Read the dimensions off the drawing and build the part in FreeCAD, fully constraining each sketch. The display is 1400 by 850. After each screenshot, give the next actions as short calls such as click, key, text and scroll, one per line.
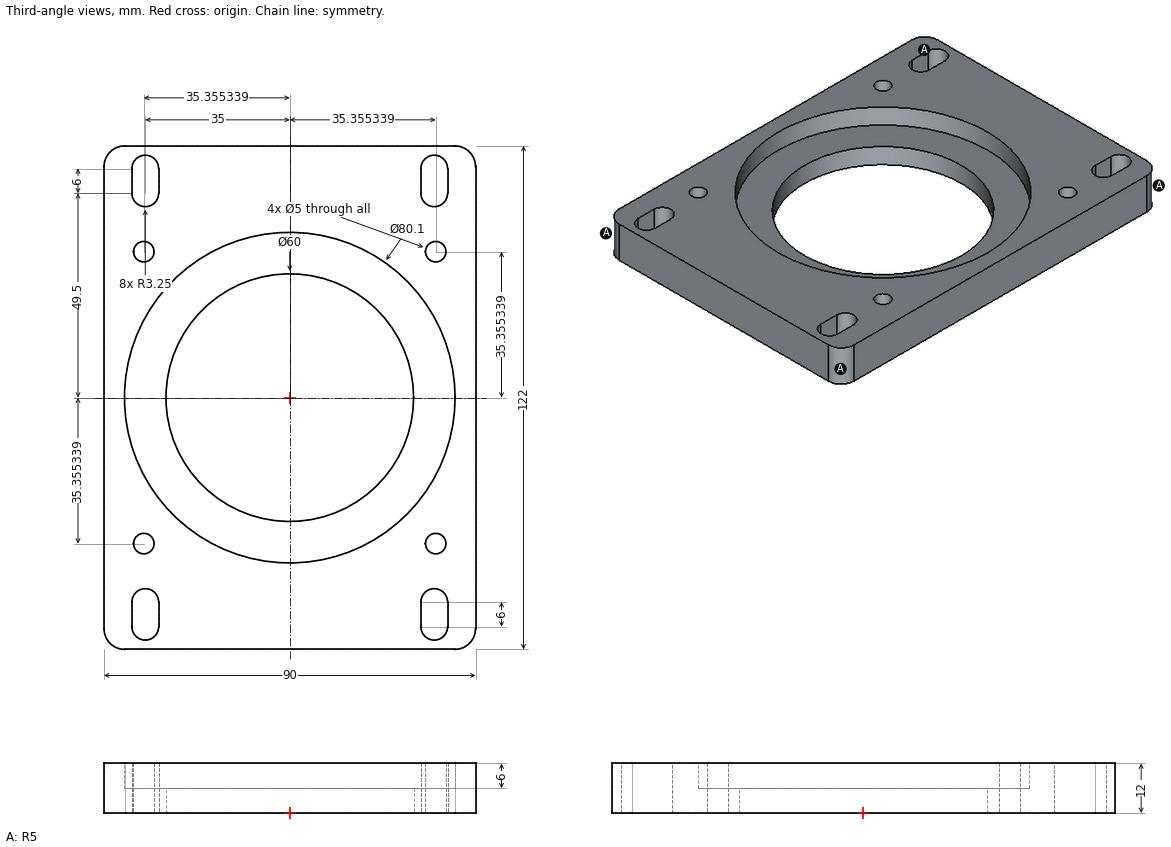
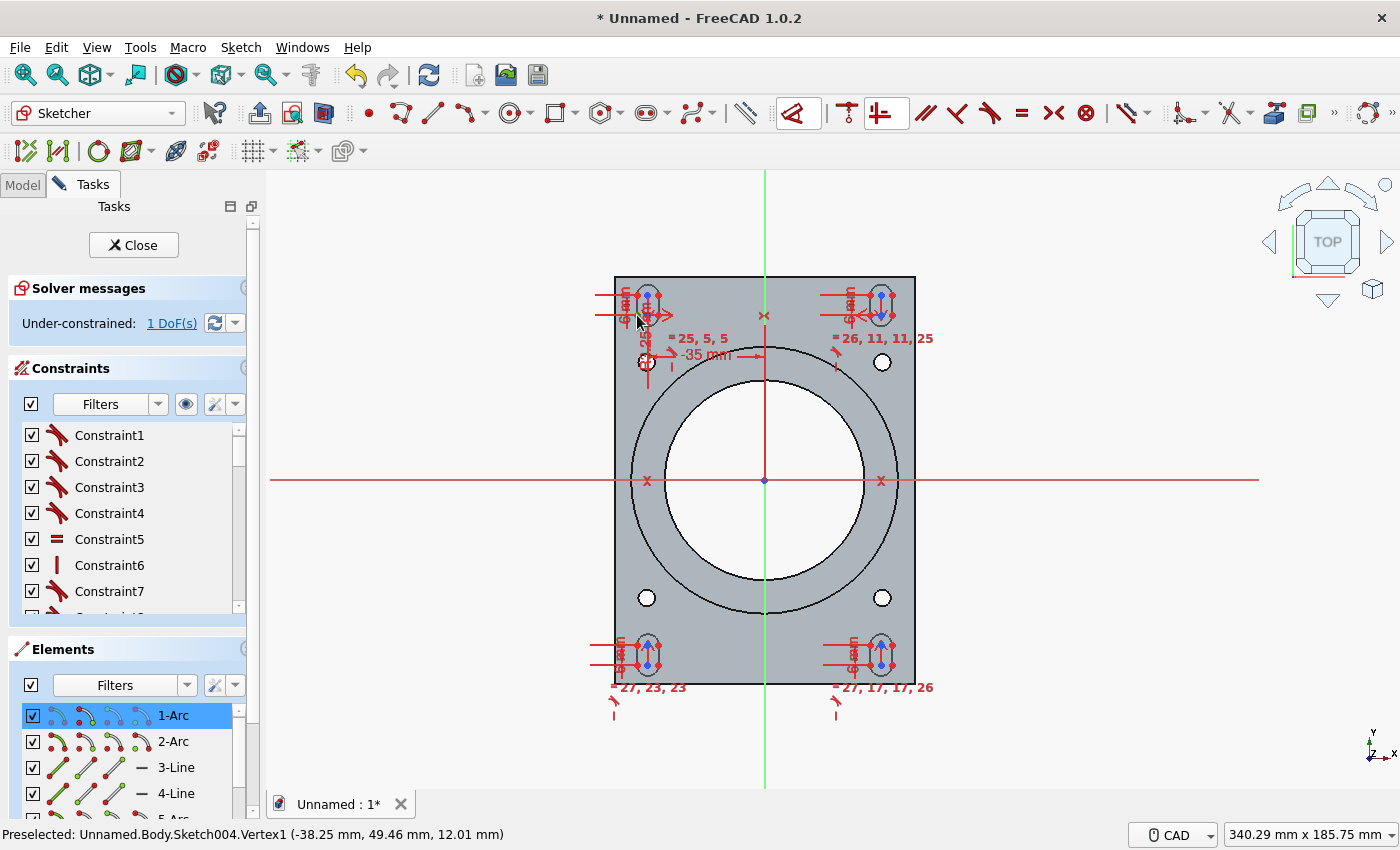
click(816, 114)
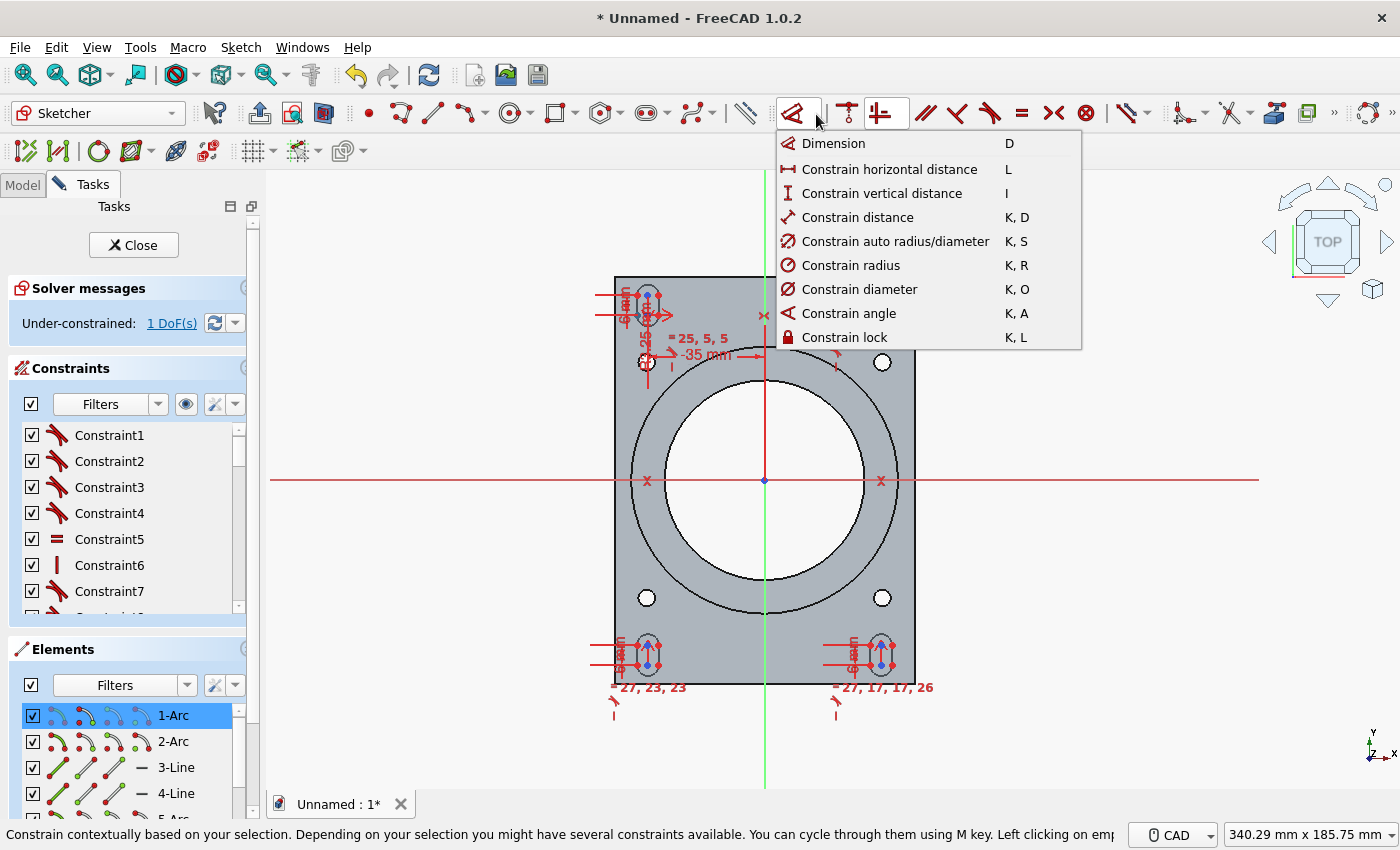
click(929, 193)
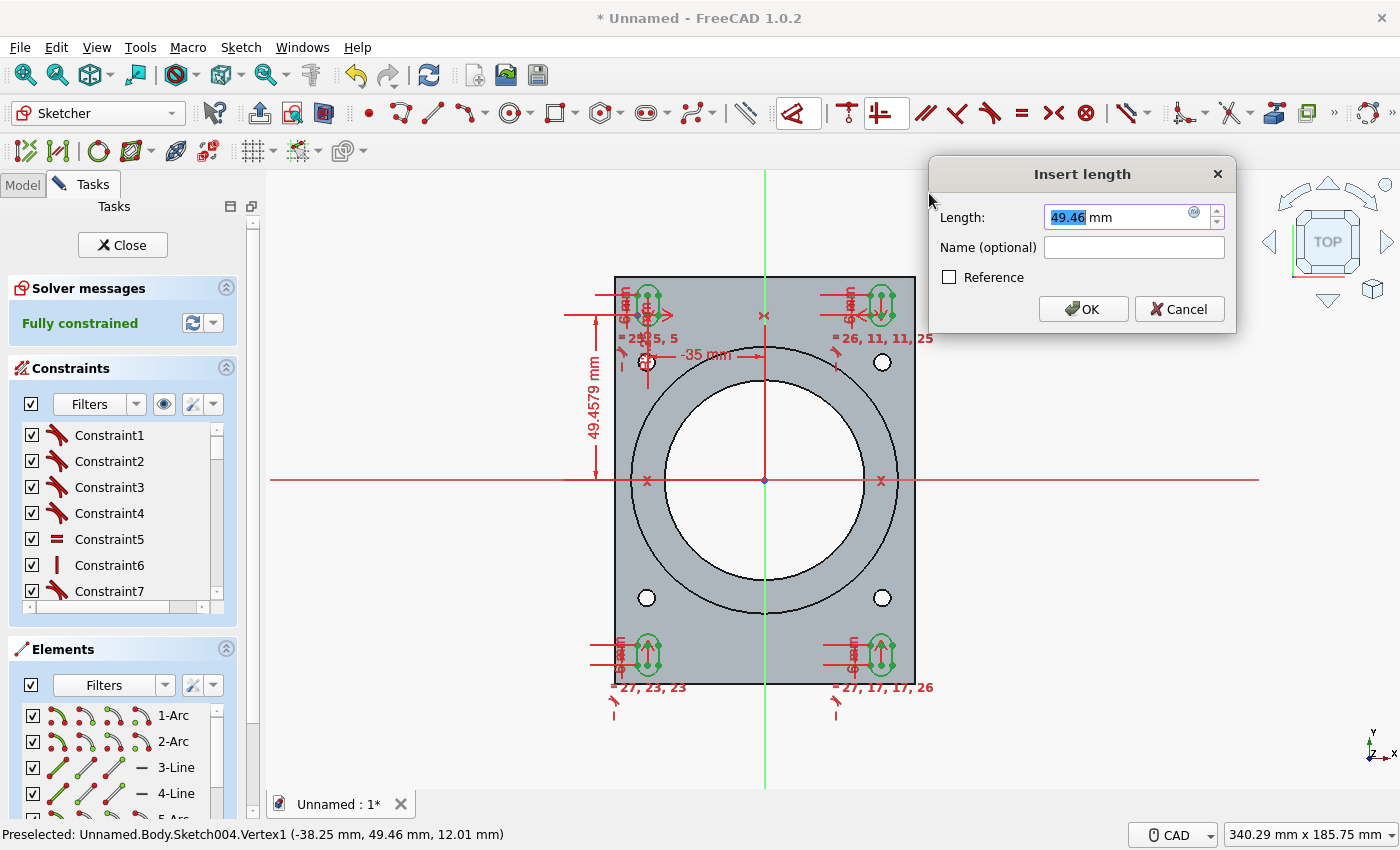
text(49.5)
key(Return)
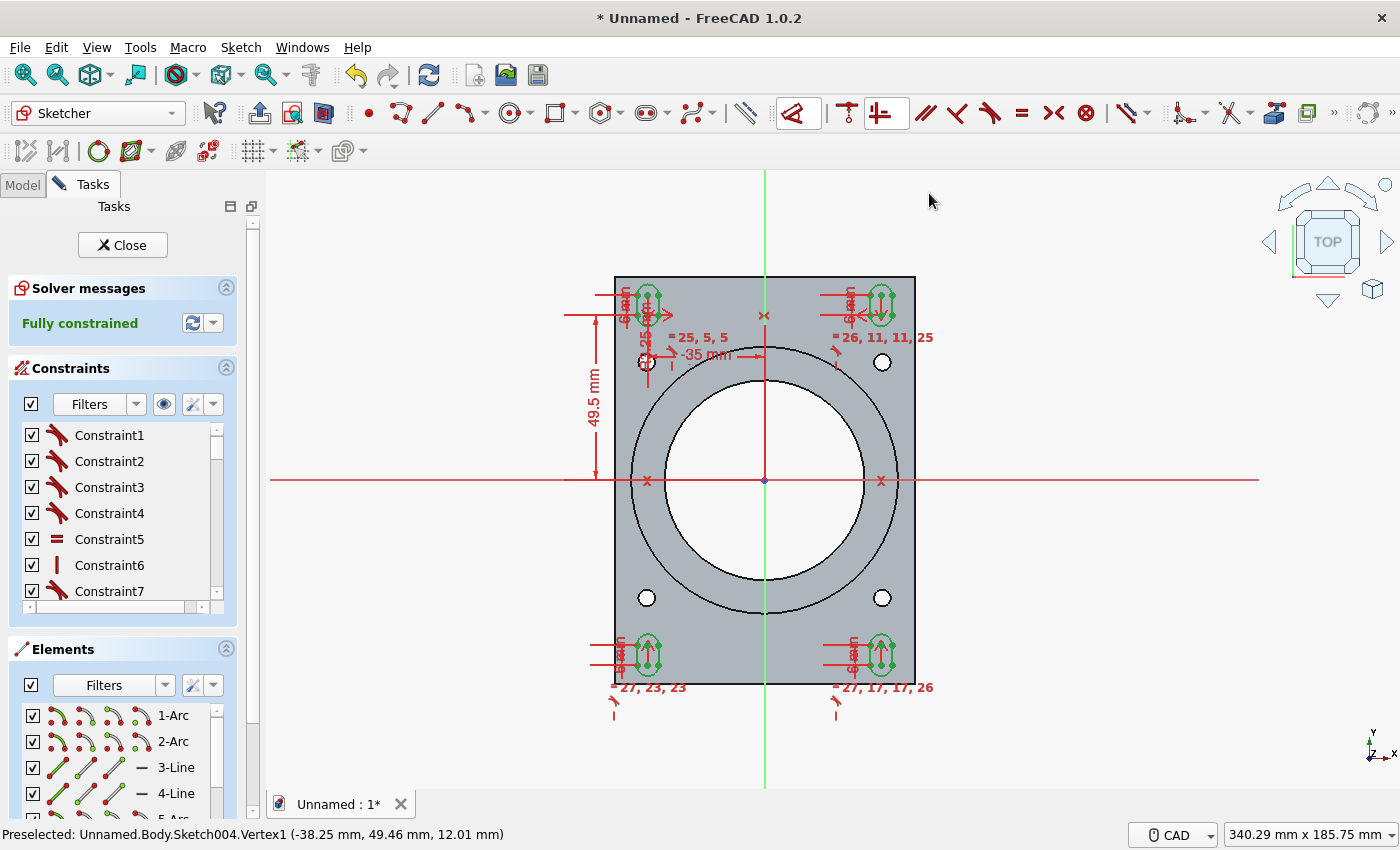
click(123, 245)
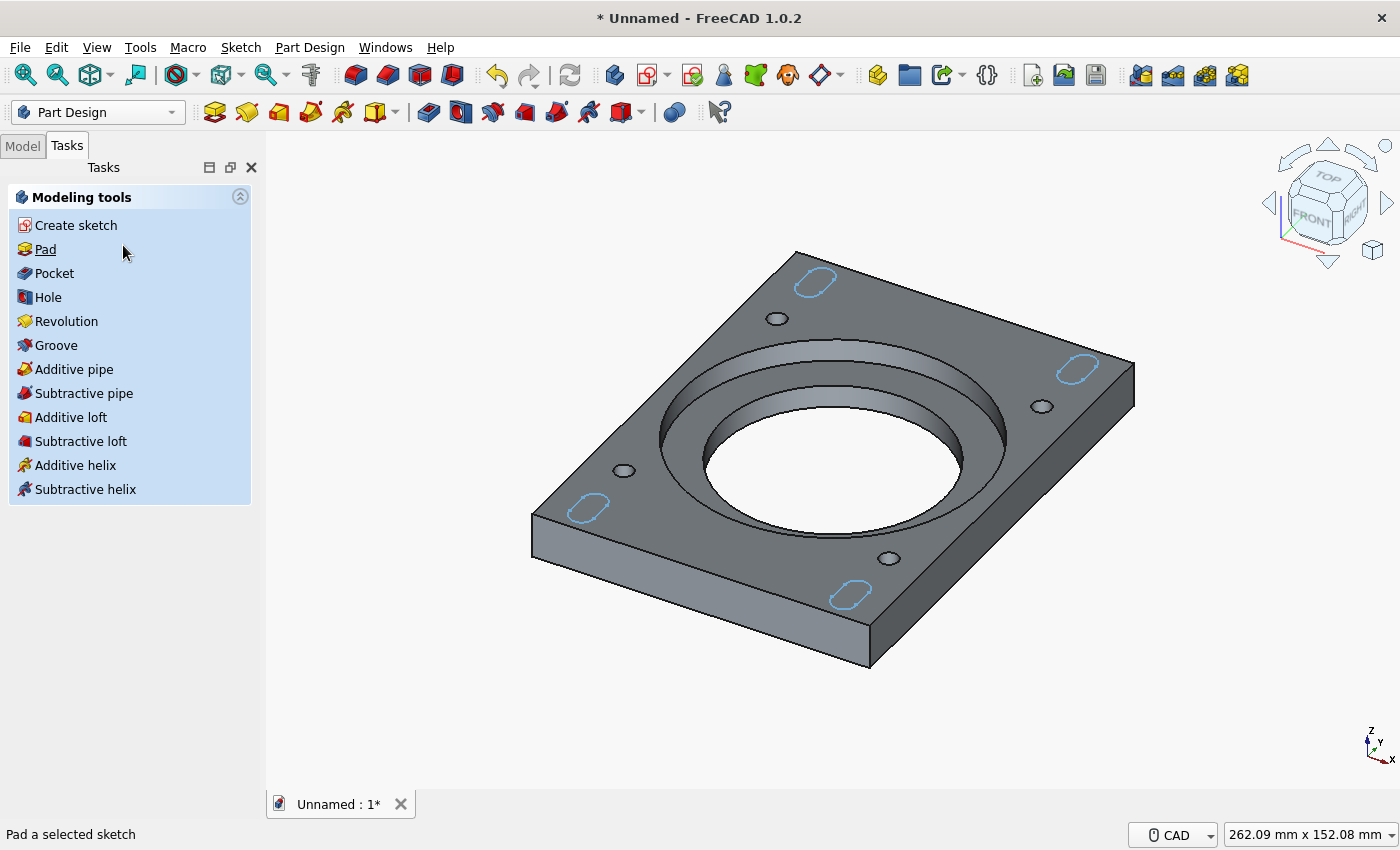
click(430, 112)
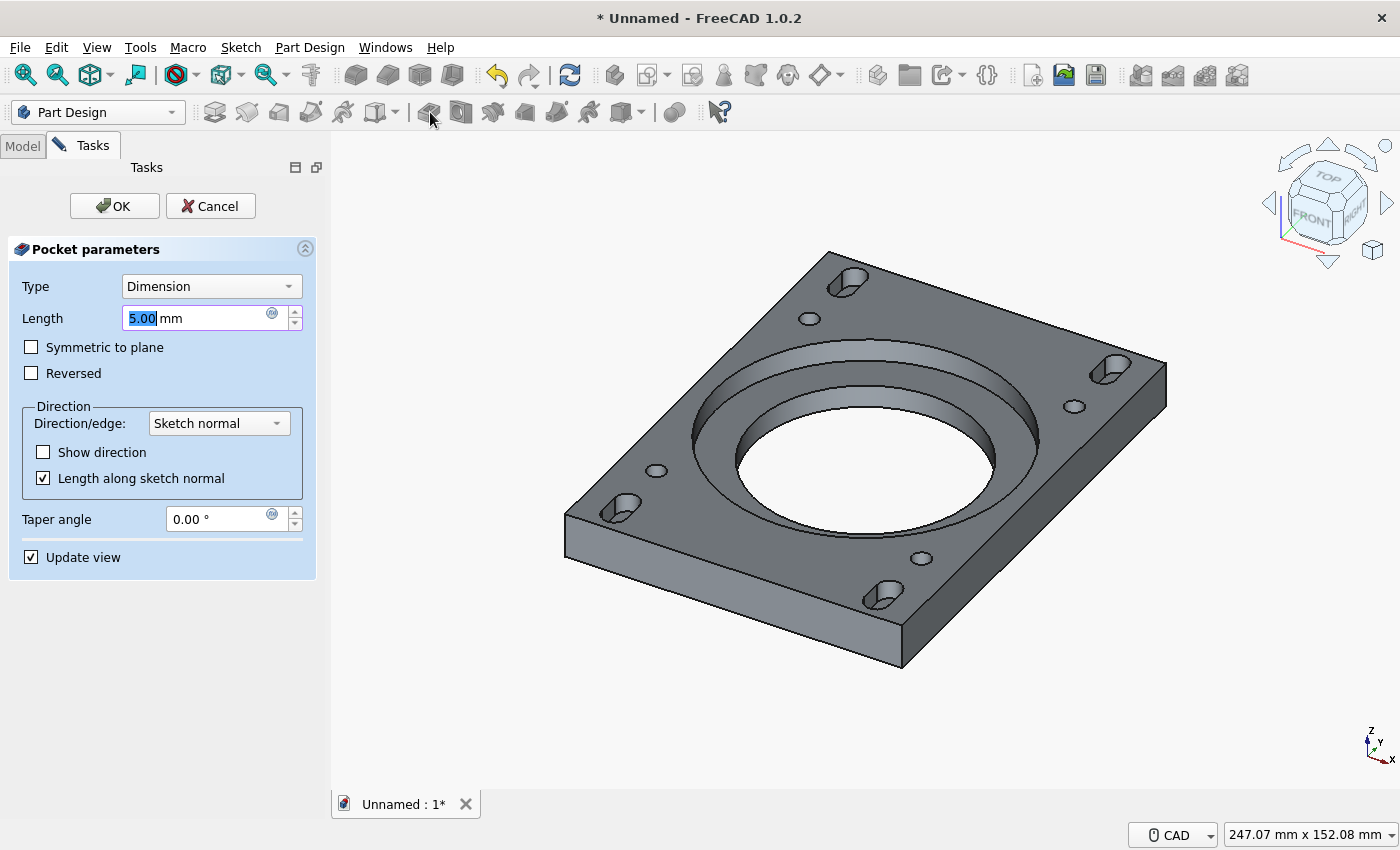
click(212, 286)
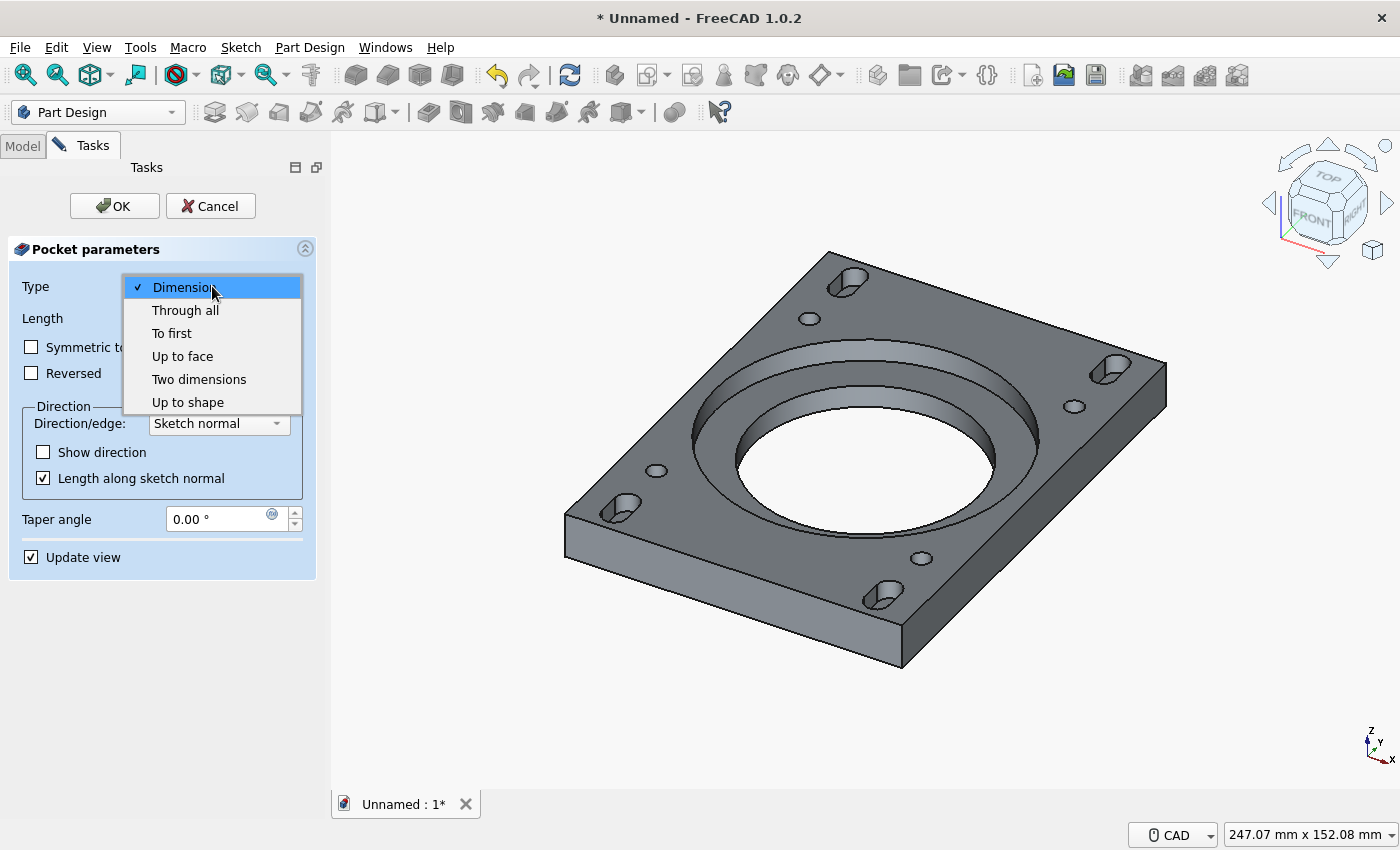
click(212, 310)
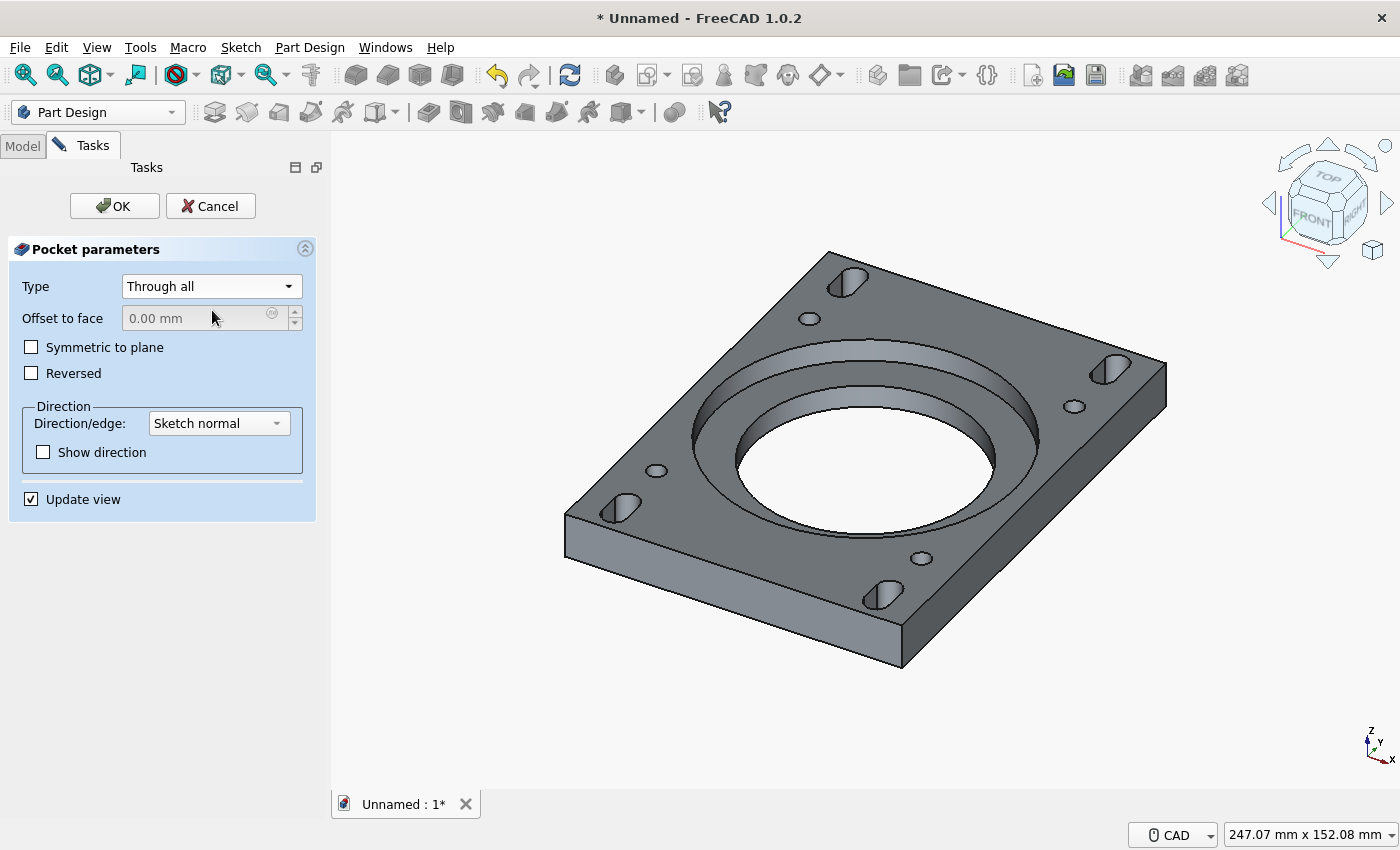
click(115, 206)